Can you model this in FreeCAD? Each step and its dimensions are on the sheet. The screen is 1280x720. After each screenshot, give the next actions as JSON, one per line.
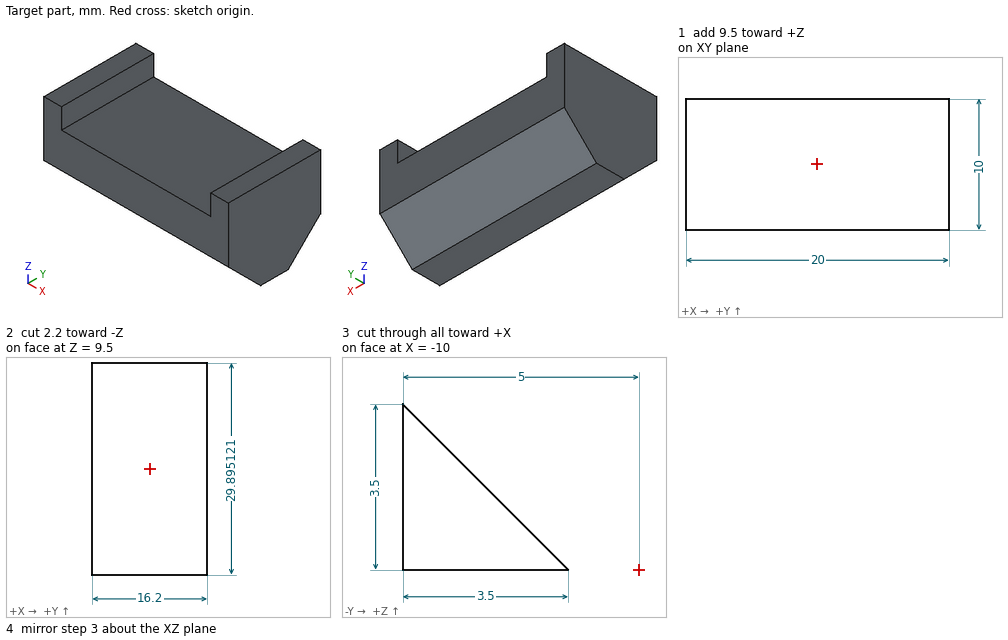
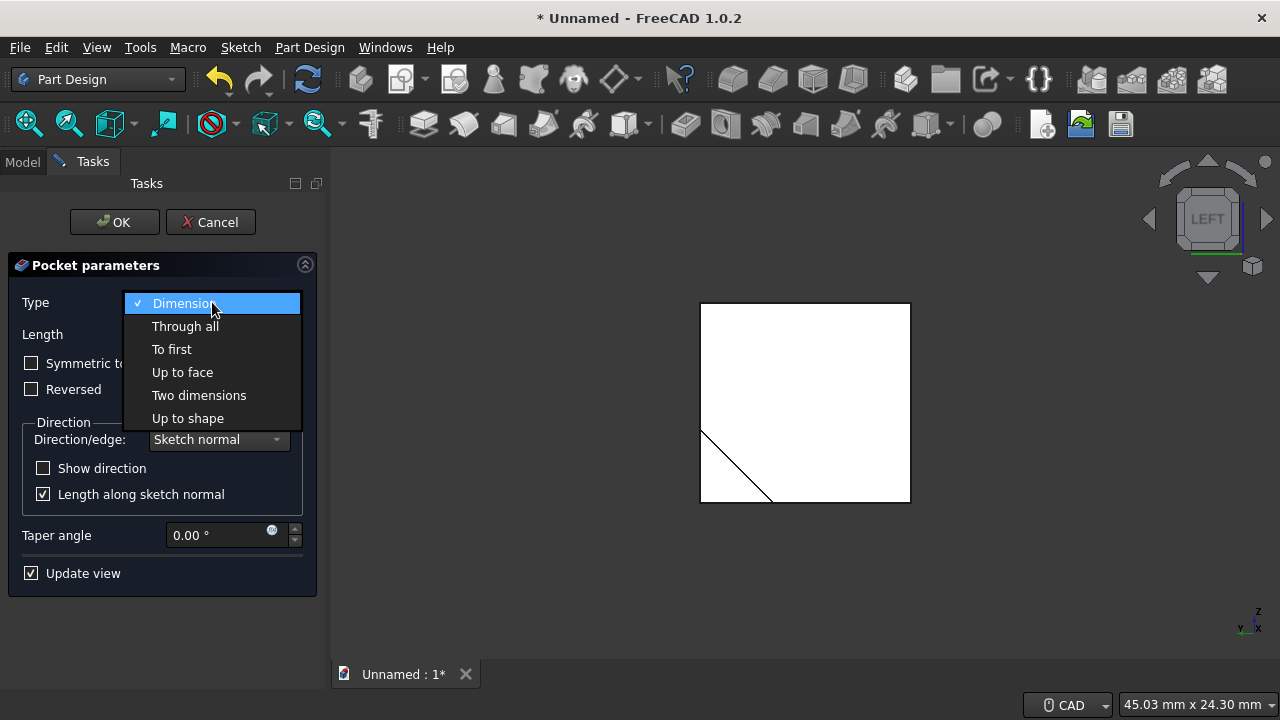
{"action": "left_click", "coordinate": [212, 326]}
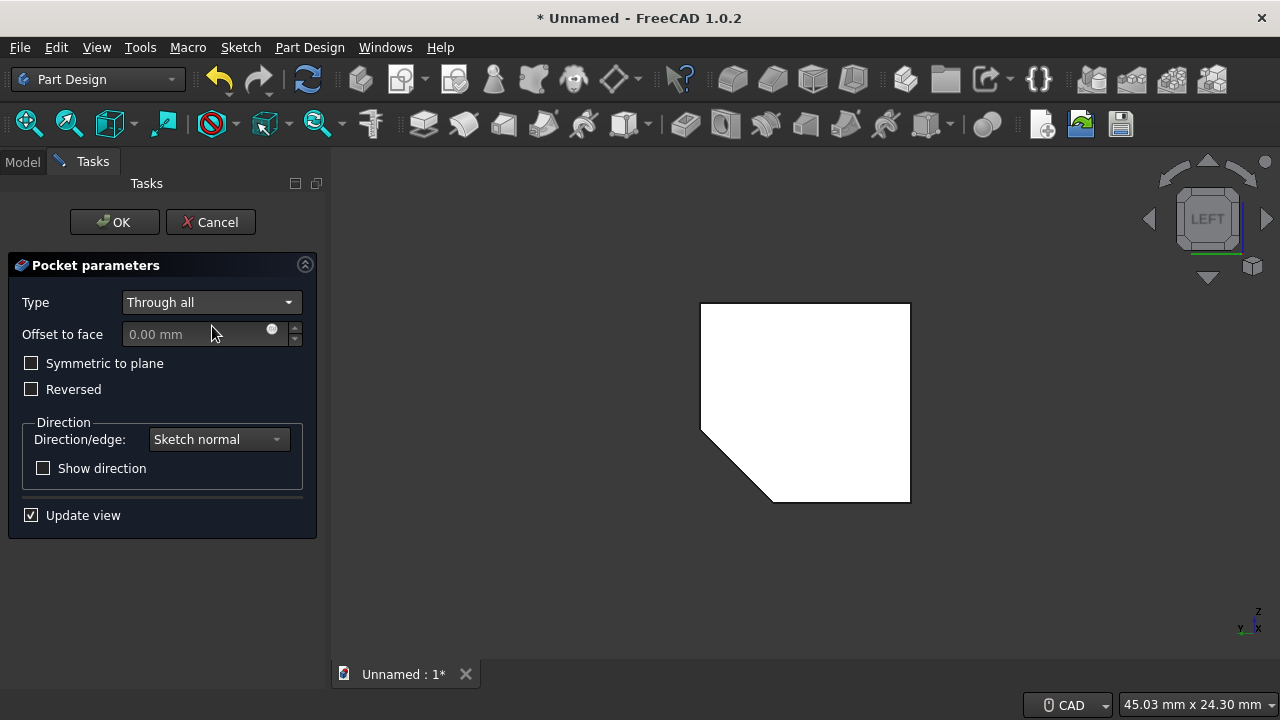
{"action": "left_click", "coordinate": [115, 222]}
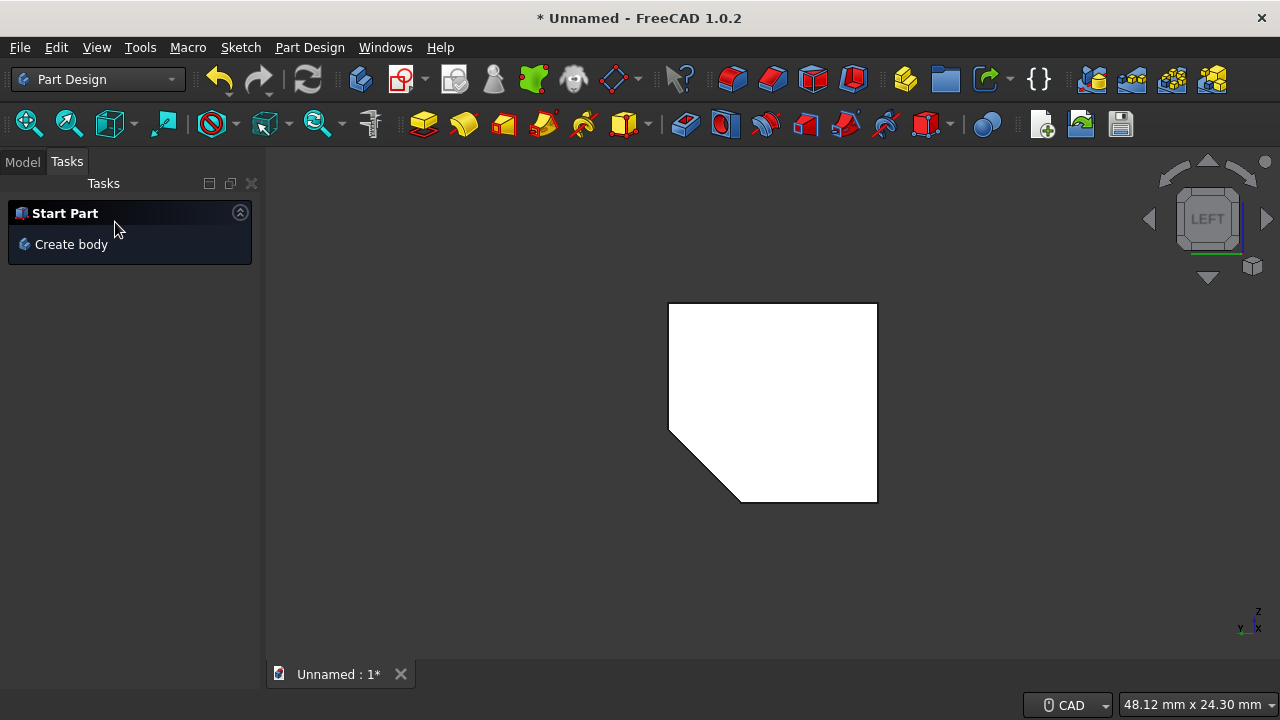
{"action": "key", "text": "v f"}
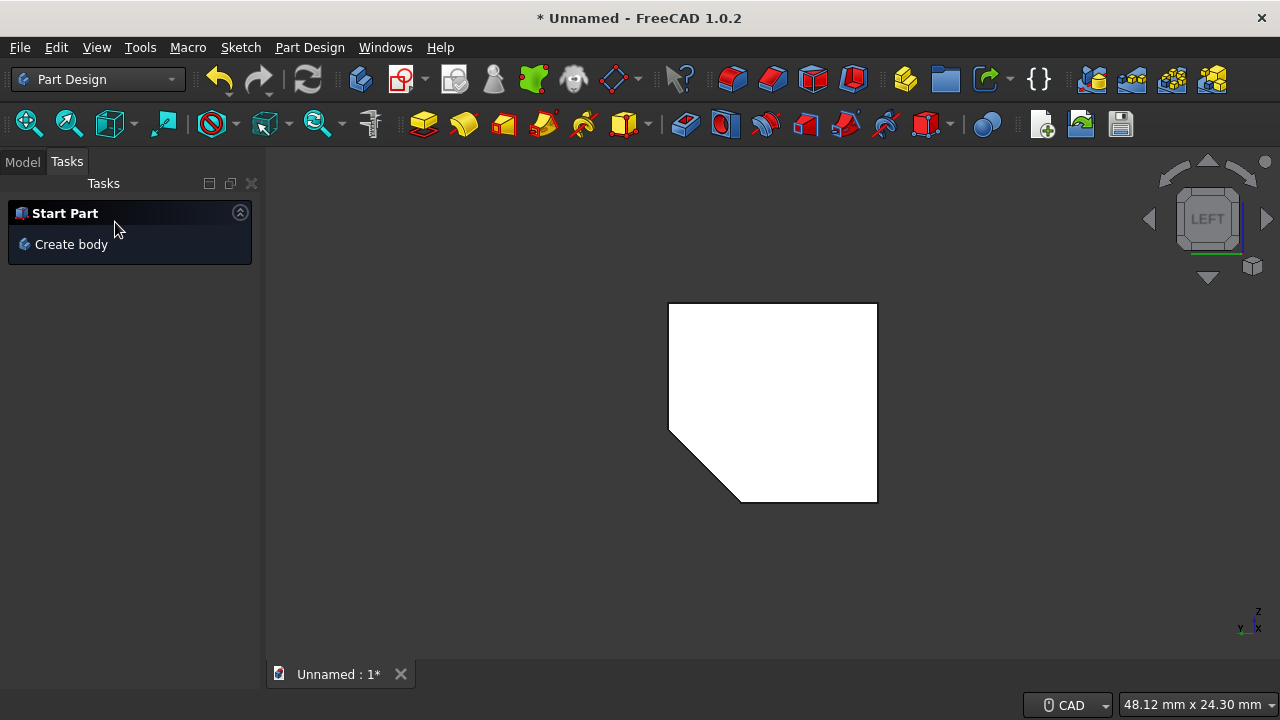
{"action": "left_click", "coordinate": [23, 161]}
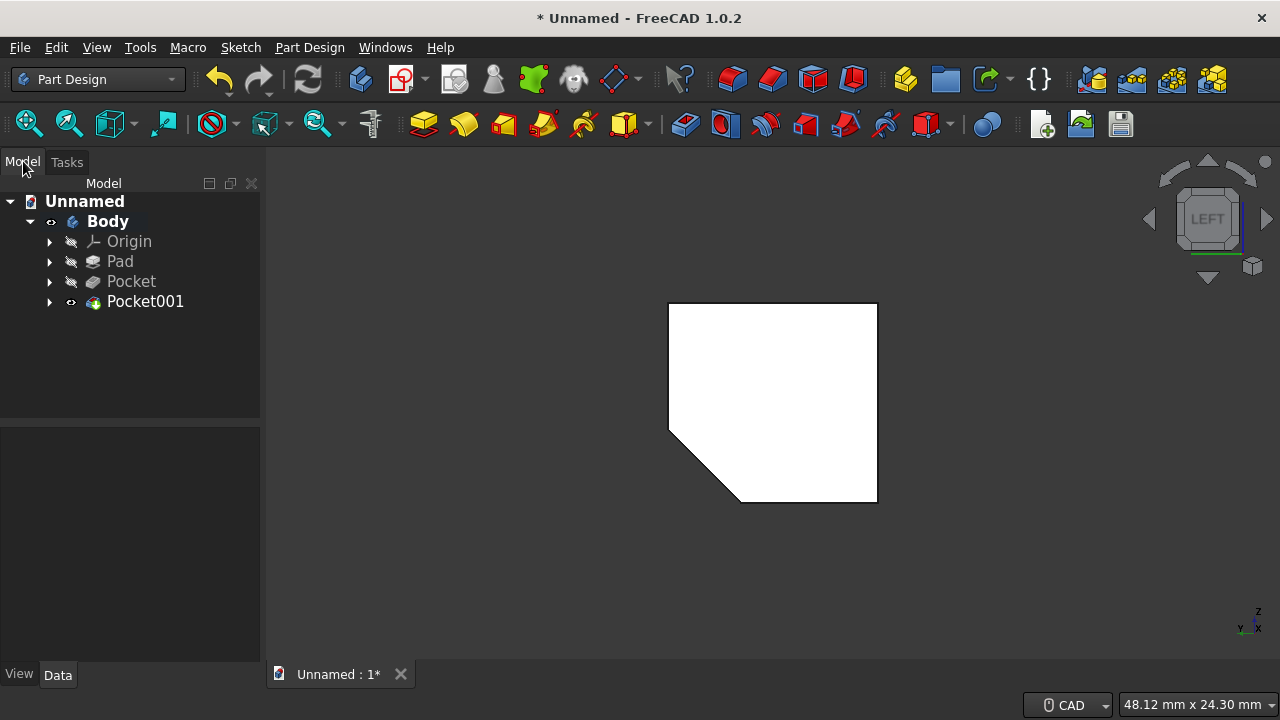
{"action": "left_click", "coordinate": [116, 302]}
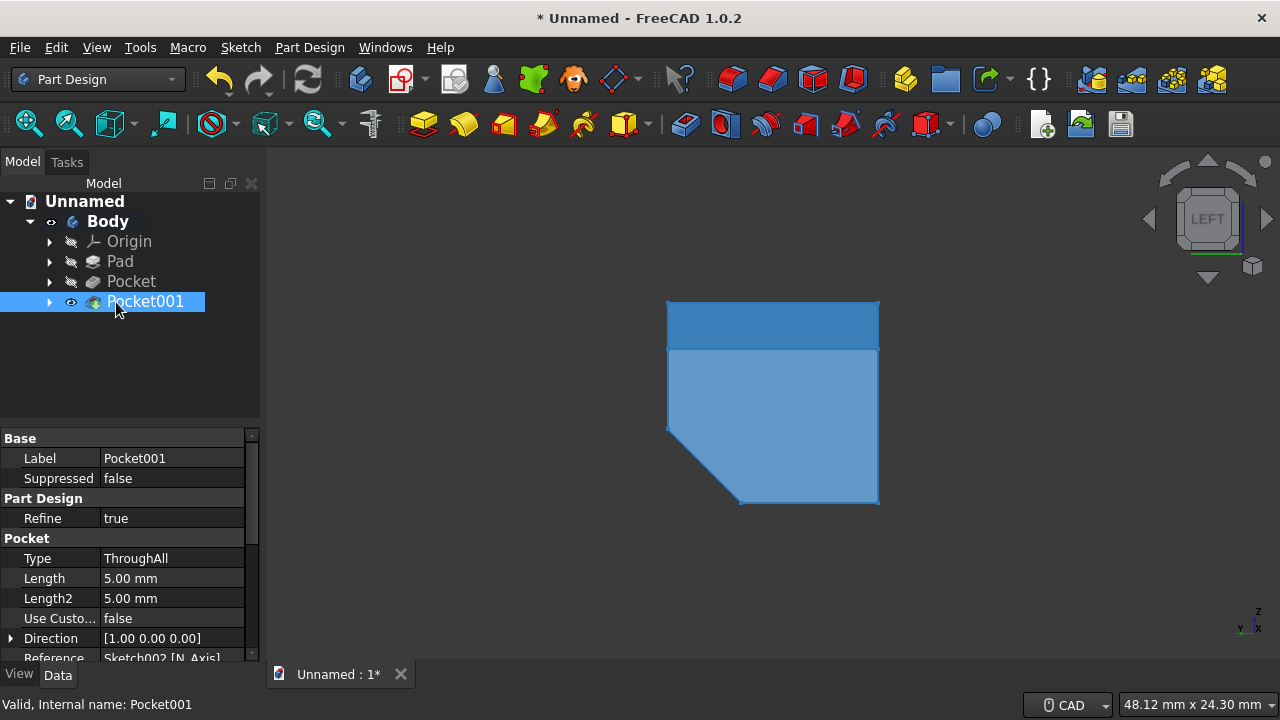
{"action": "left_click", "coordinate": [1092, 80]}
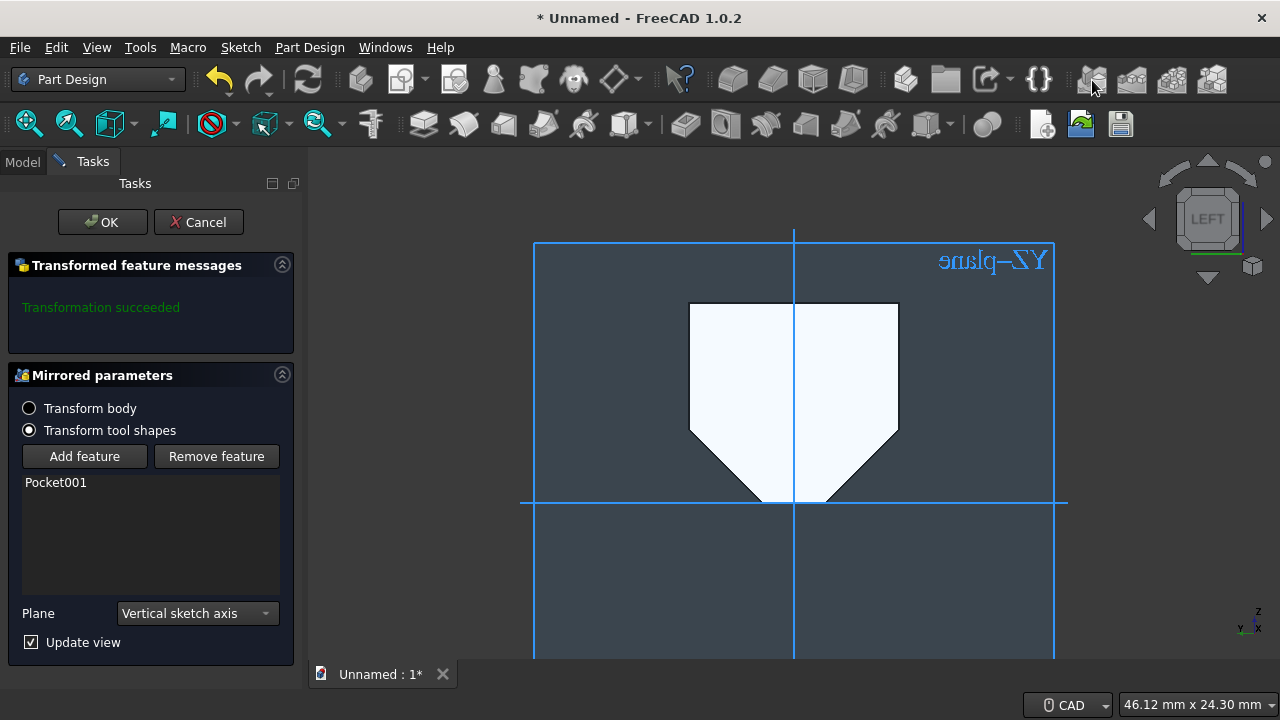
{"action": "left_click", "coordinate": [198, 614]}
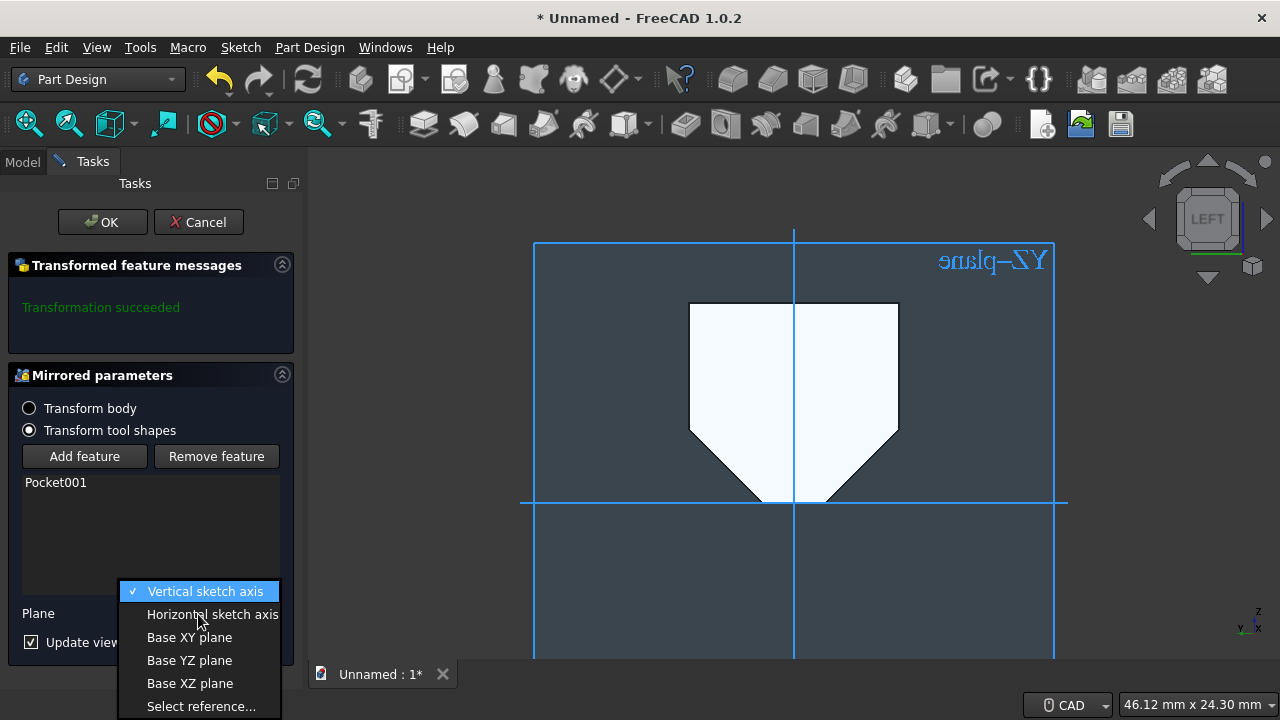
{"action": "left_click", "coordinate": [198, 684]}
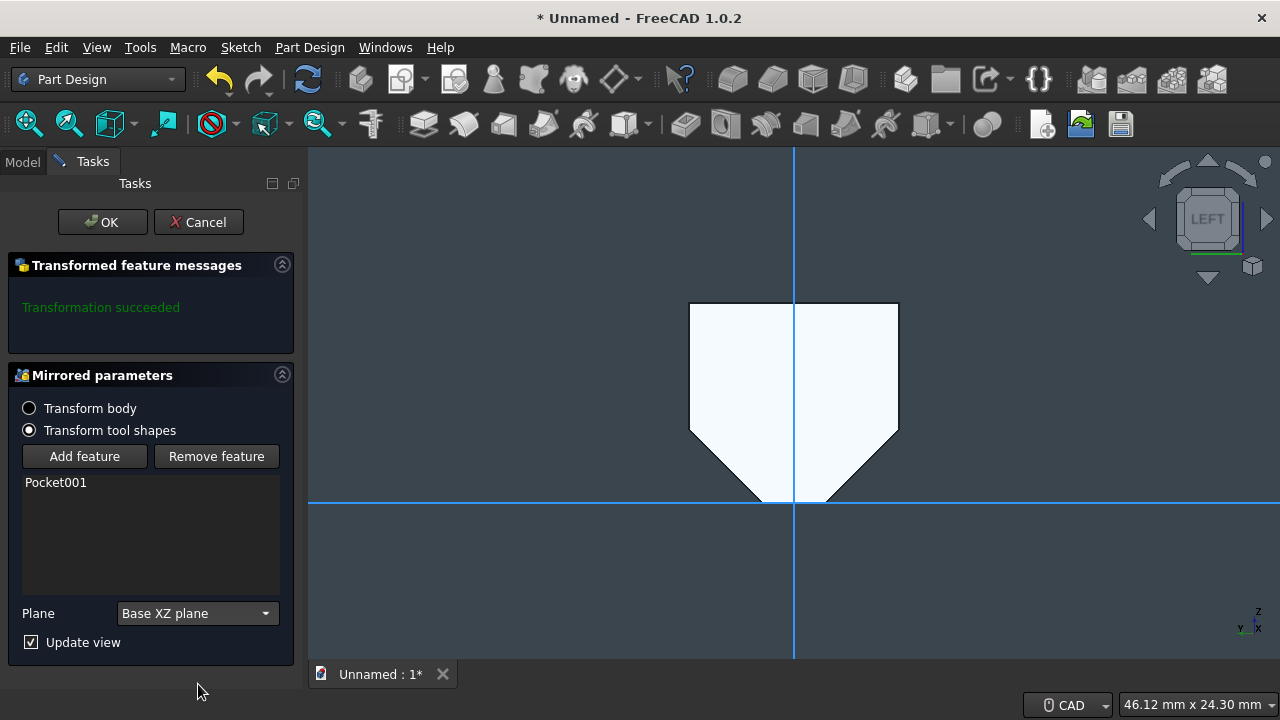
{"action": "left_click", "coordinate": [103, 222]}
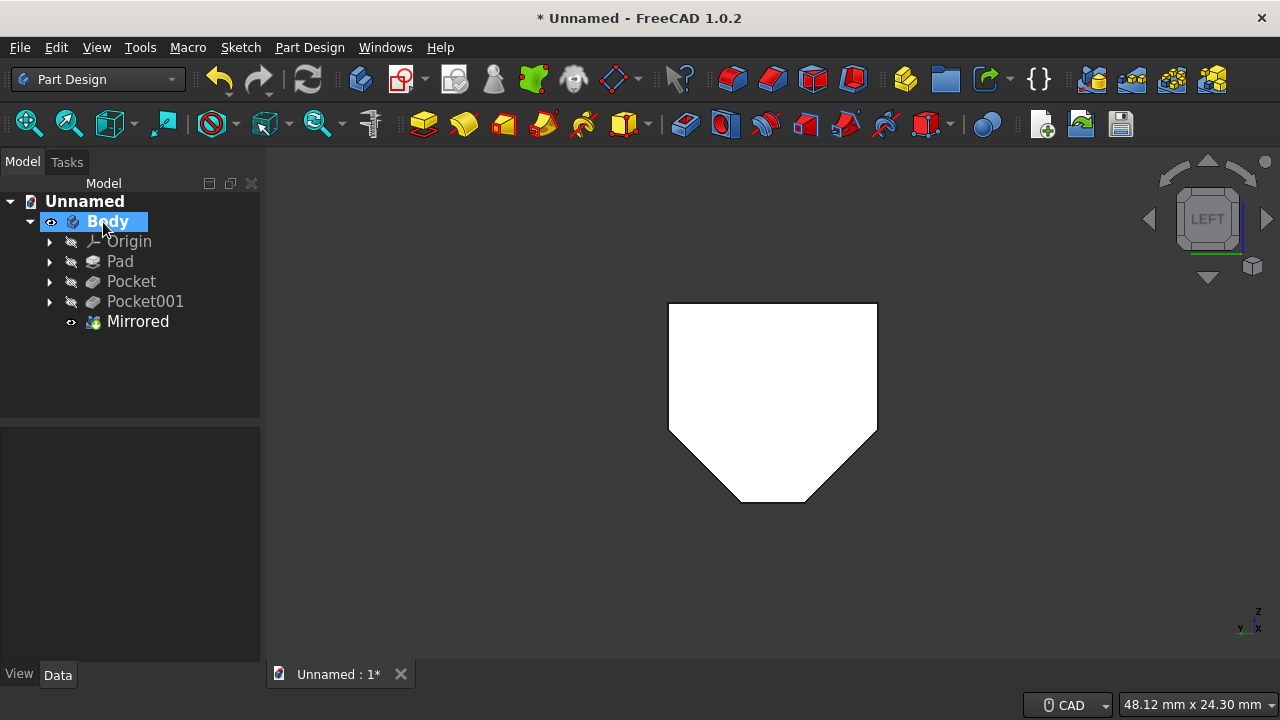
{"action": "key", "text": "0"}